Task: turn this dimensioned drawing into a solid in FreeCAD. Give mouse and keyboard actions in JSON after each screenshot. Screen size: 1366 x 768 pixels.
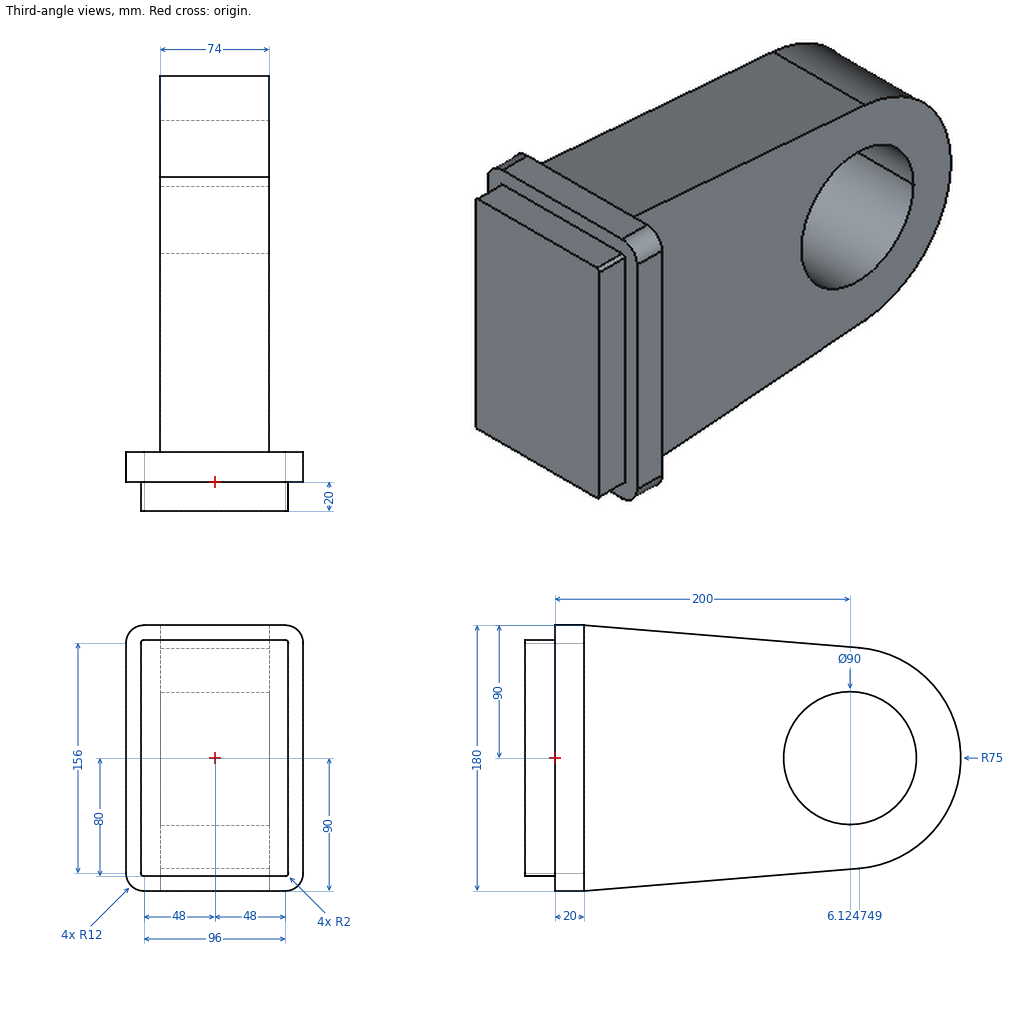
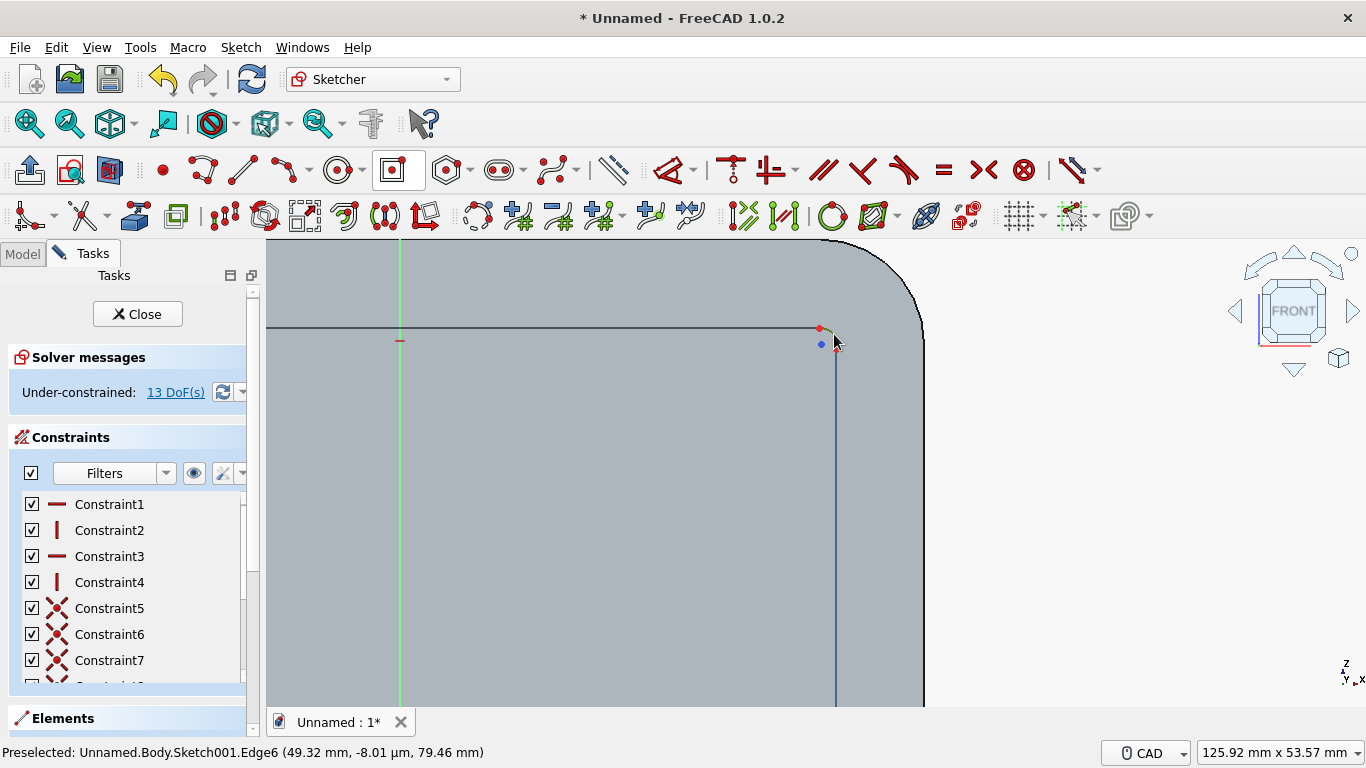
{"action": "key", "text": "t"}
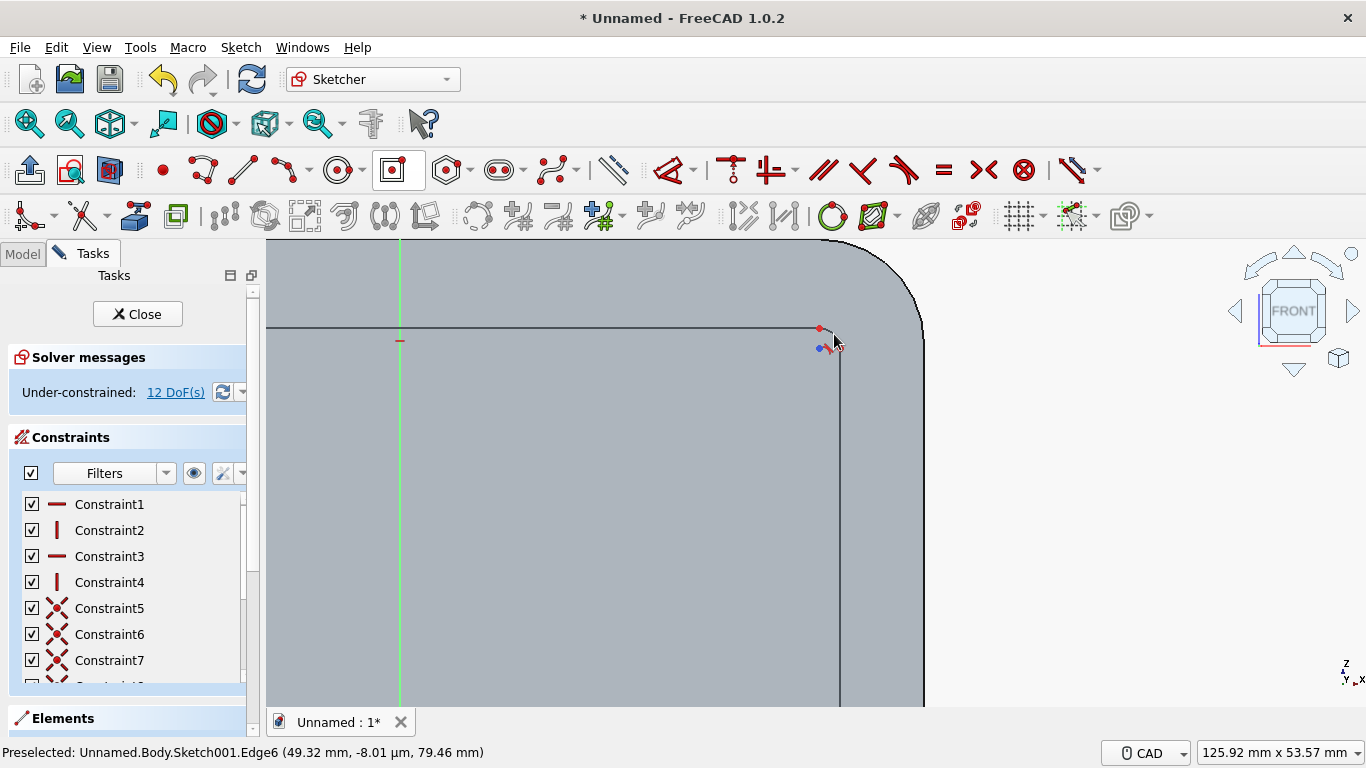
{"action": "scroll", "coordinate": [835, 333], "scroll_direction": "down", "scroll_amount": 8}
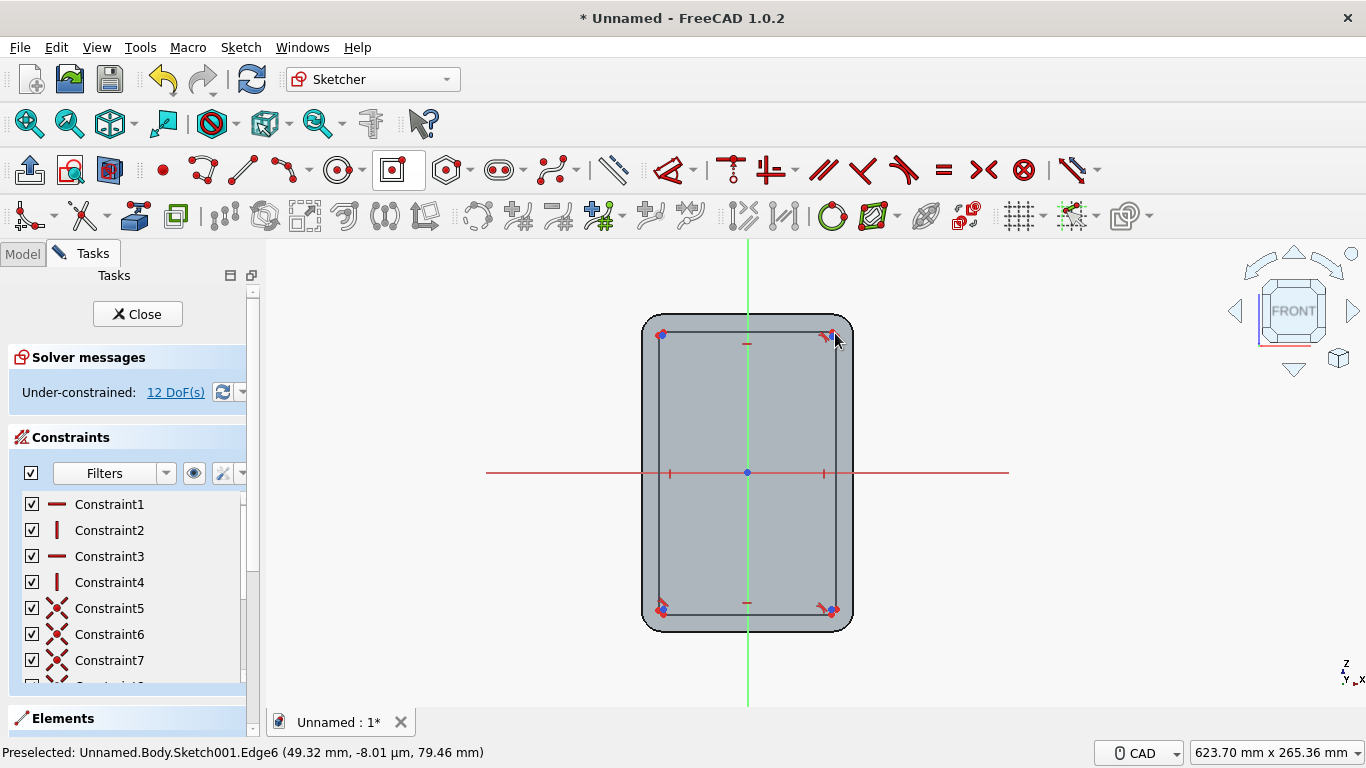
{"action": "left_click", "coordinate": [782, 332]}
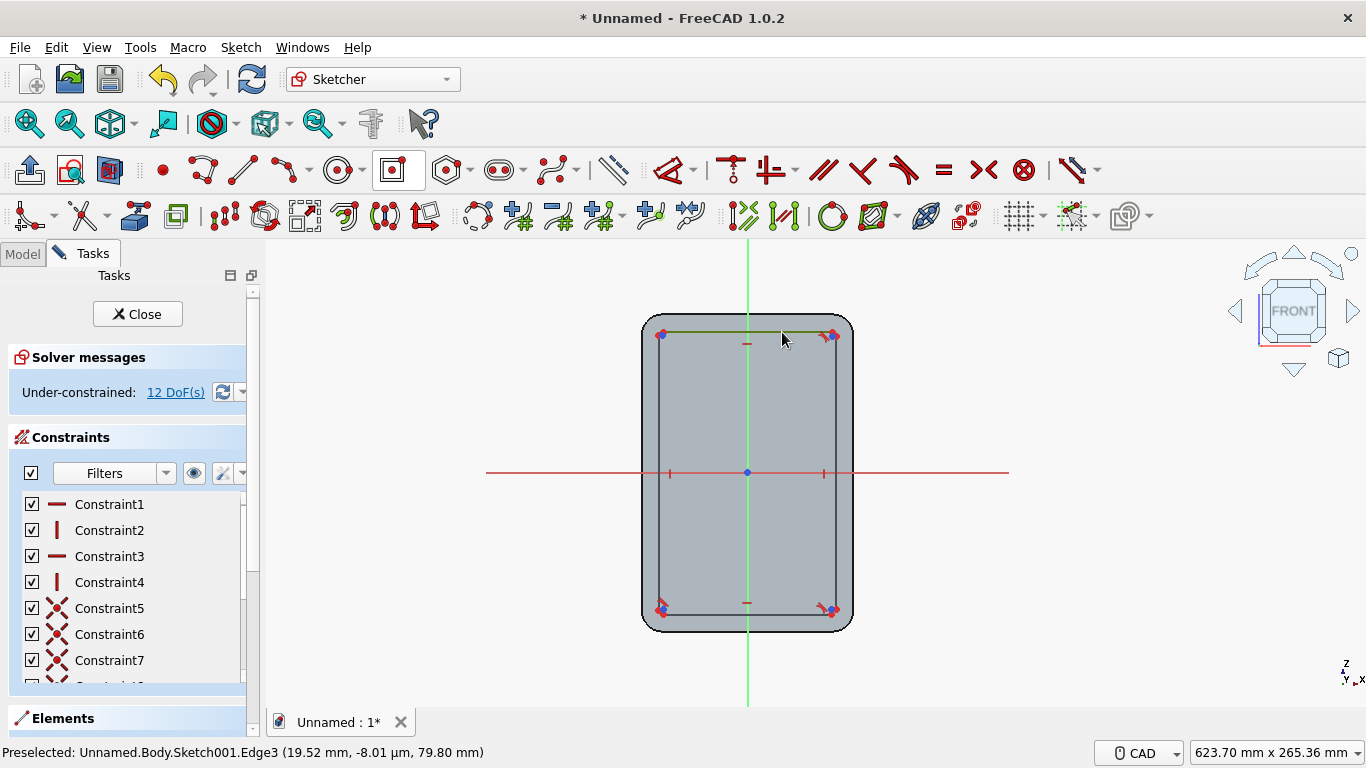
{"action": "scroll", "coordinate": [835, 333], "scroll_direction": "up", "scroll_amount": 8}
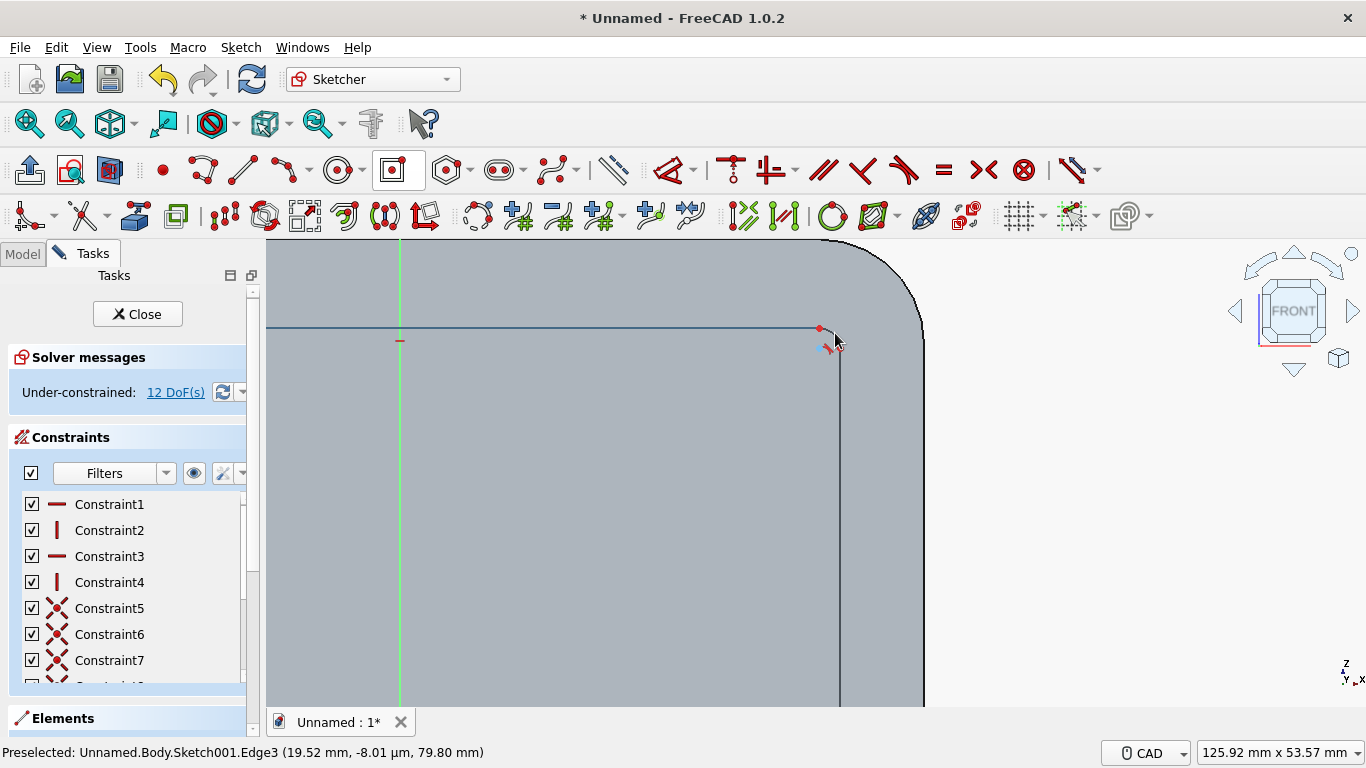
{"action": "left_click", "coordinate": [834, 335]}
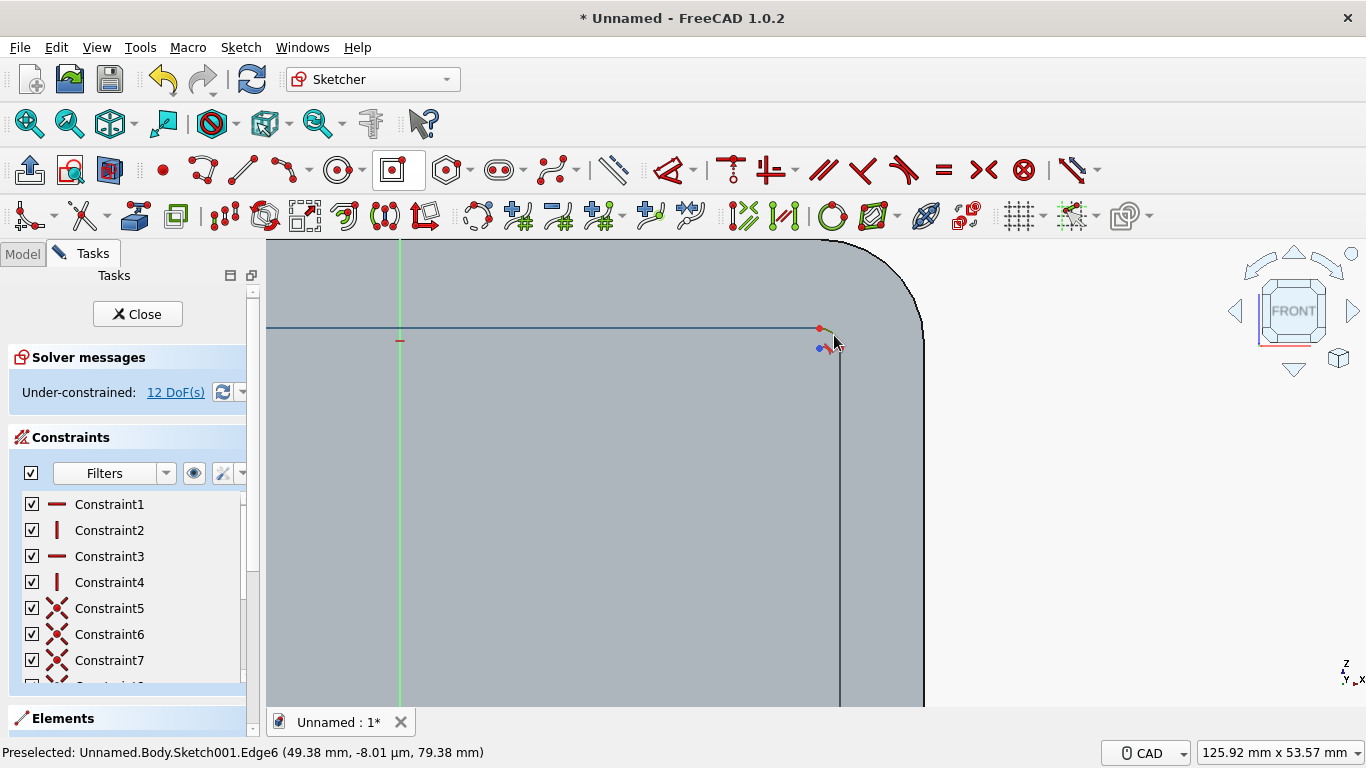
{"action": "key", "text": "t"}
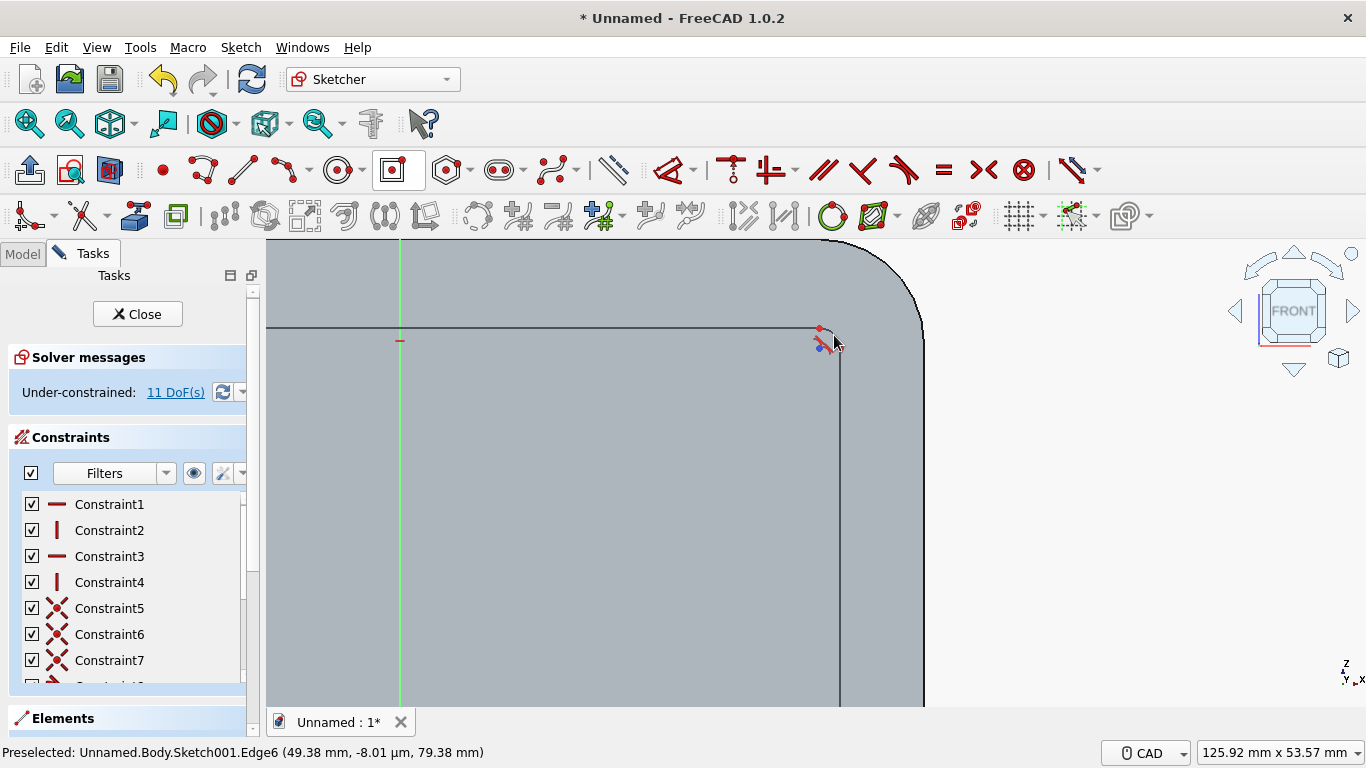
{"action": "scroll", "coordinate": [835, 333], "scroll_direction": "down", "scroll_amount": 8}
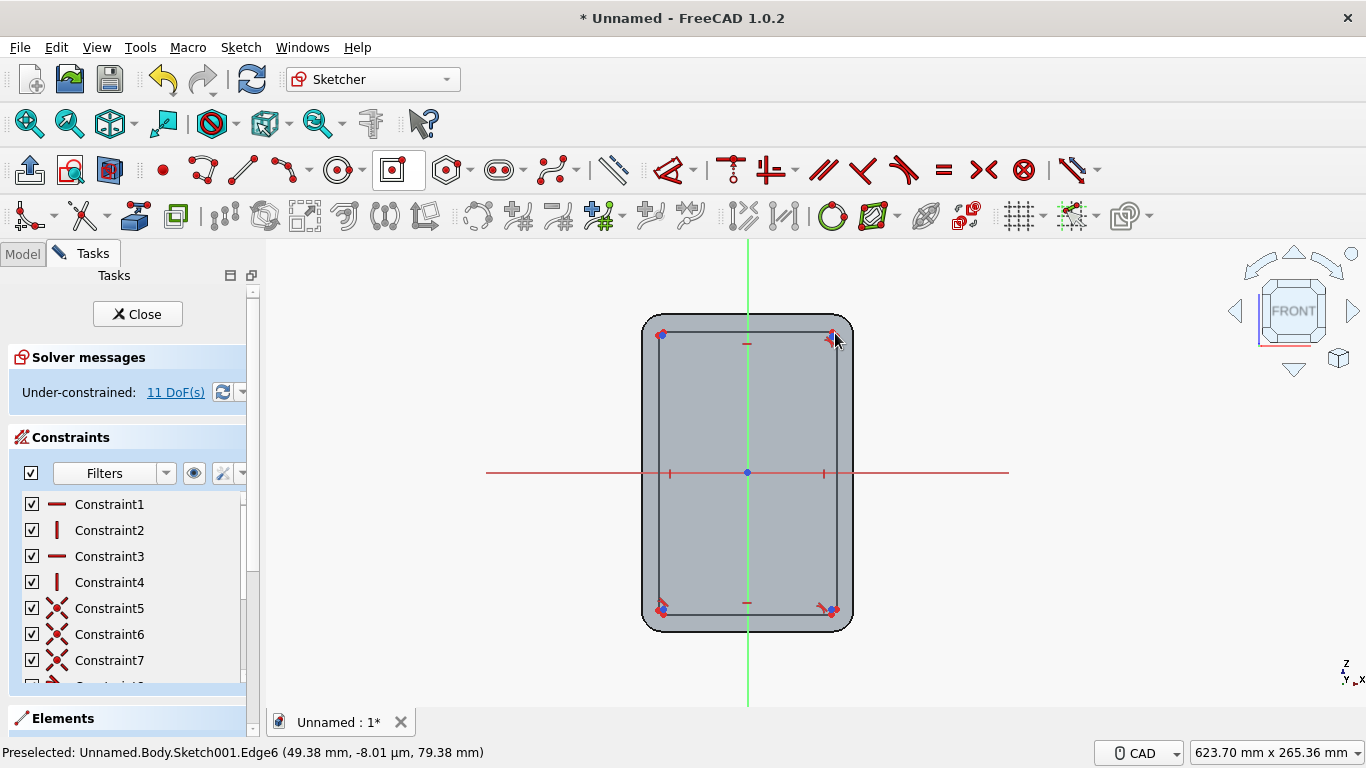
{"action": "left_click", "coordinate": [782, 332]}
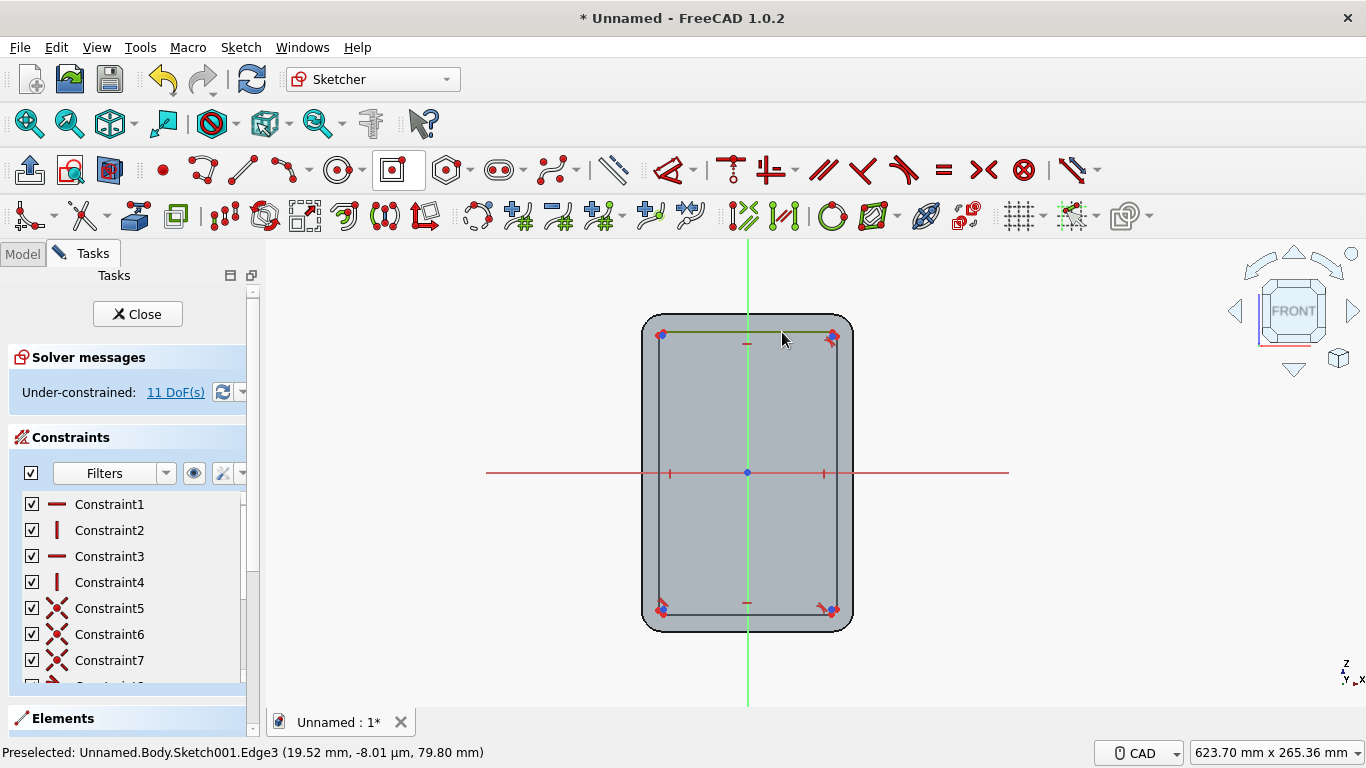
{"action": "scroll", "coordinate": [660, 333], "scroll_direction": "up", "scroll_amount": 8}